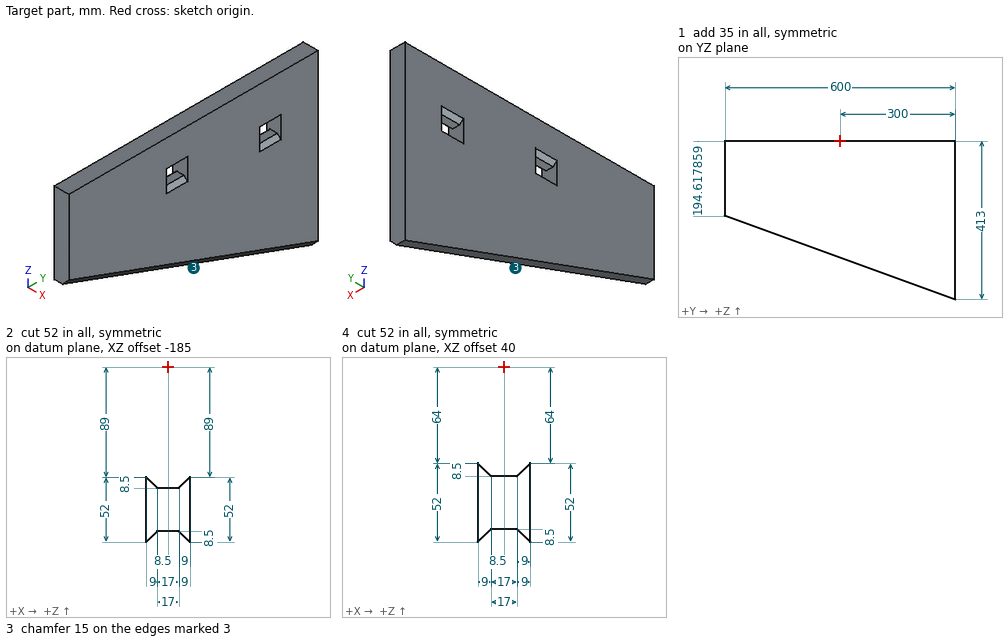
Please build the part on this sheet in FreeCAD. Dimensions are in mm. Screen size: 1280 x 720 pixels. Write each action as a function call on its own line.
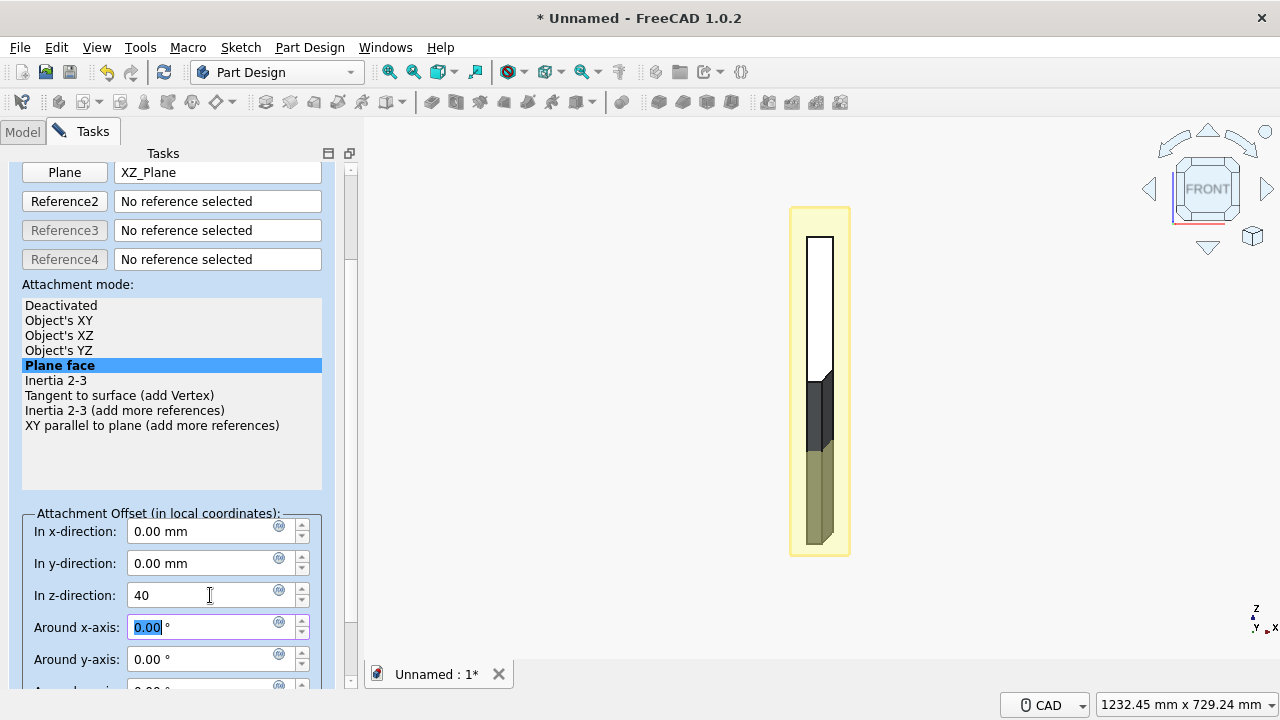
scroll(351, 426, up, 3)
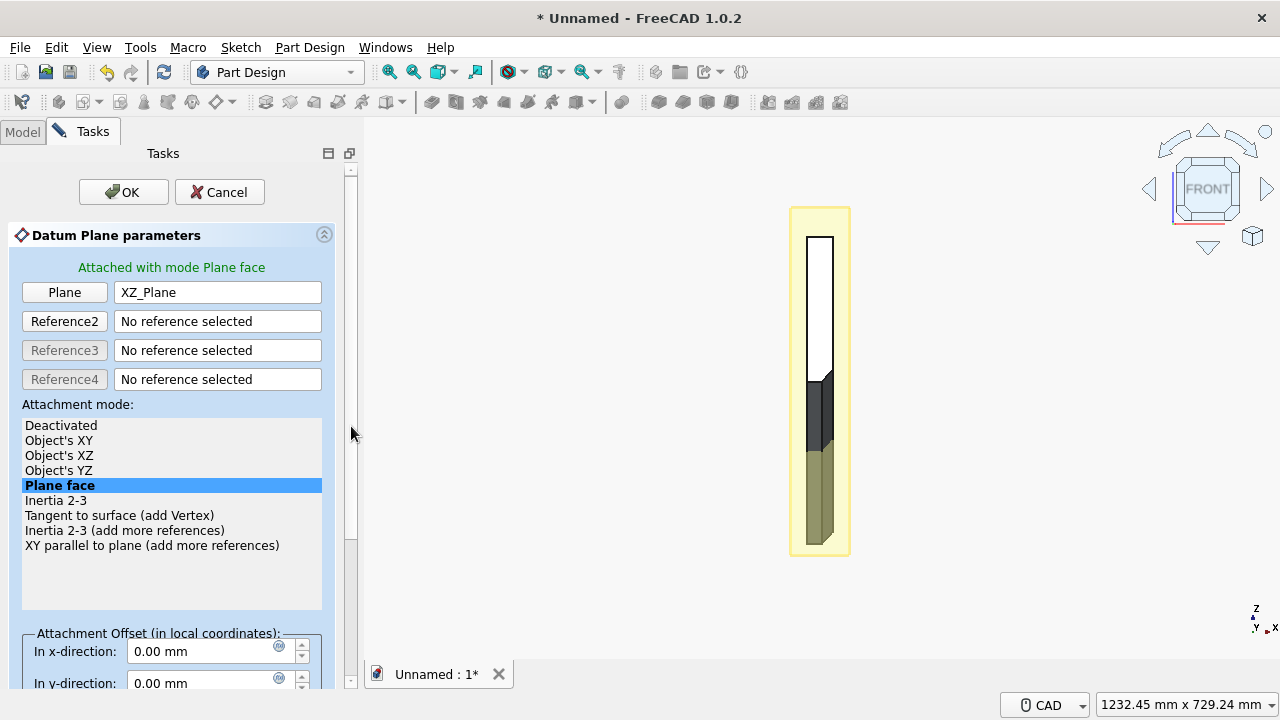
click(124, 192)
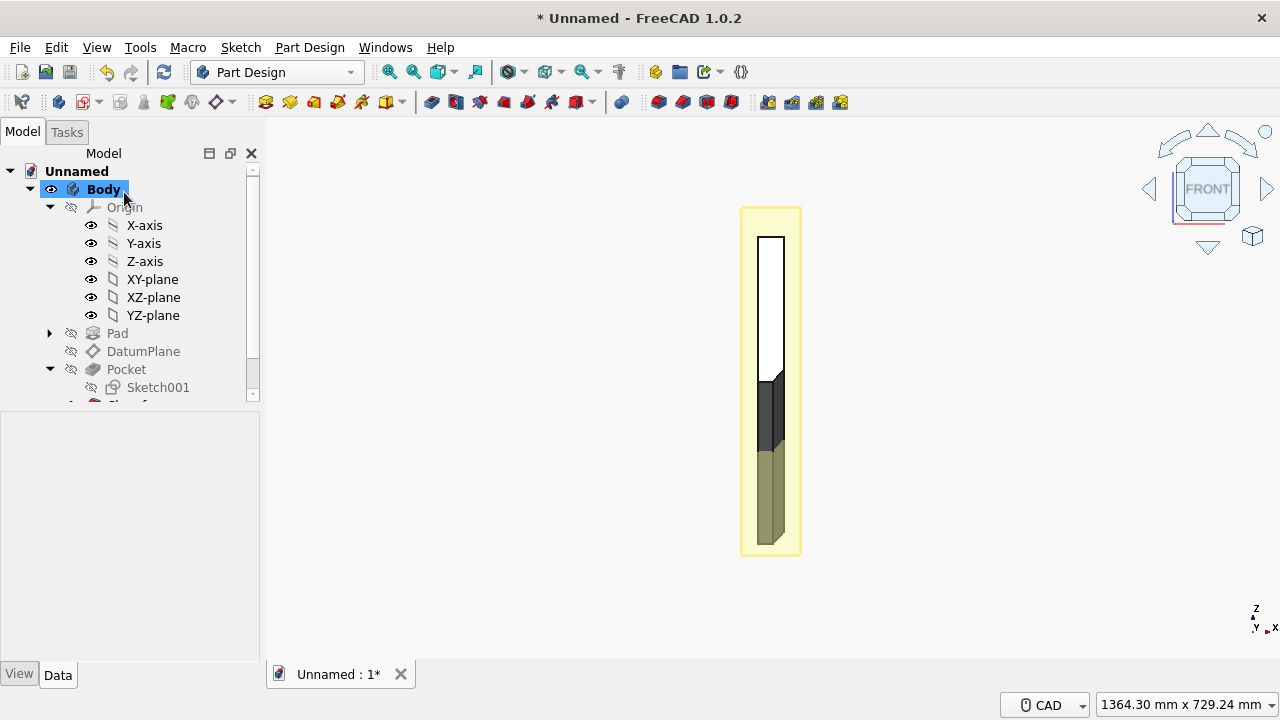
scroll(100, 275, down, 3)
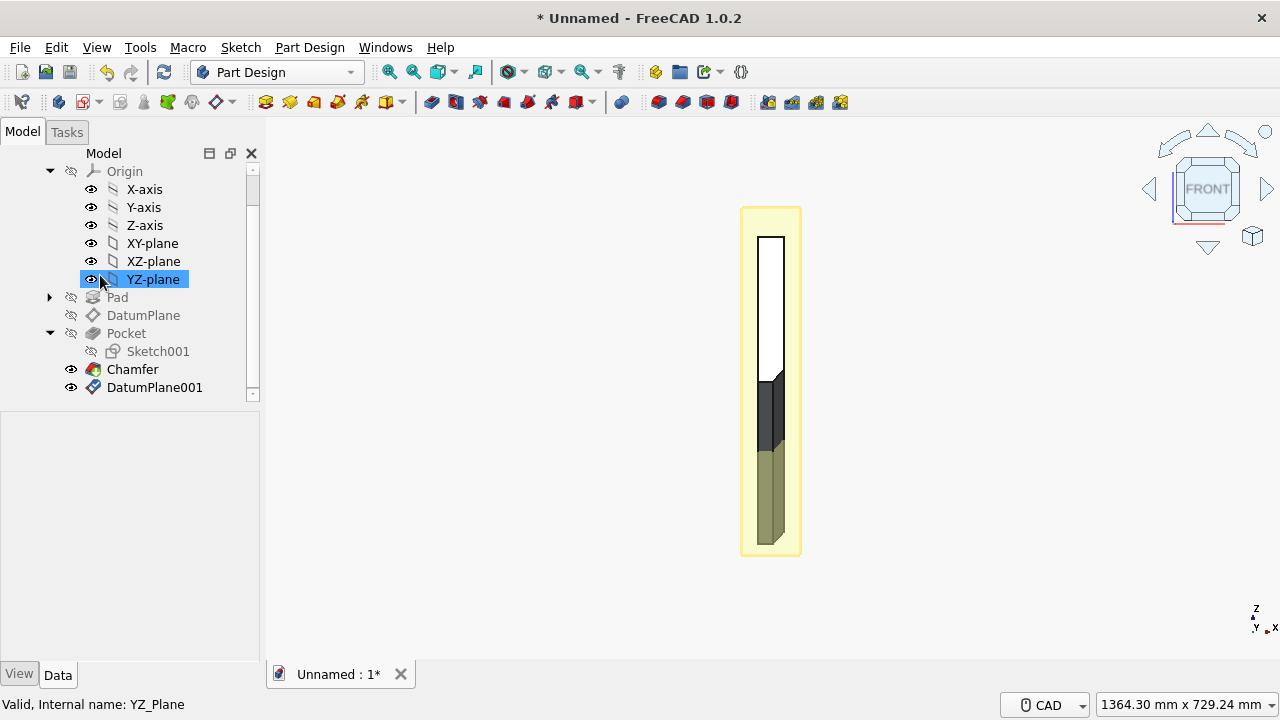
click(116, 387)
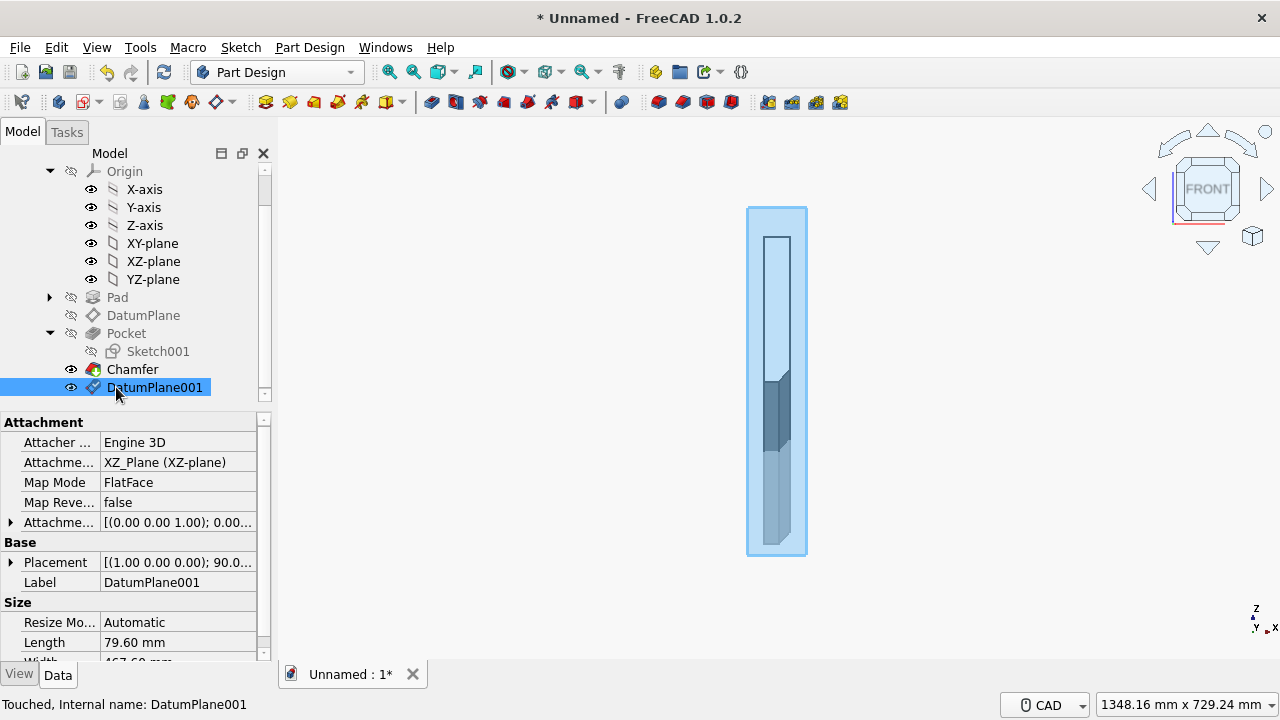
click(84, 102)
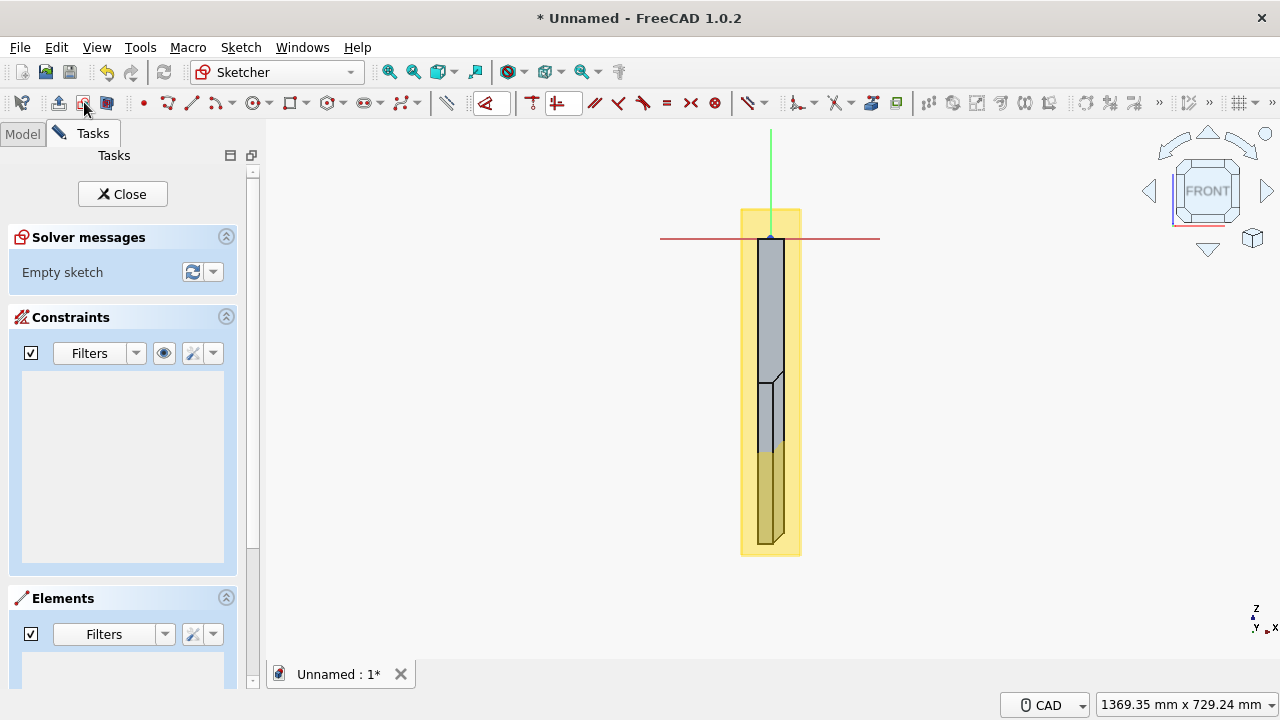
key(q)
key(s)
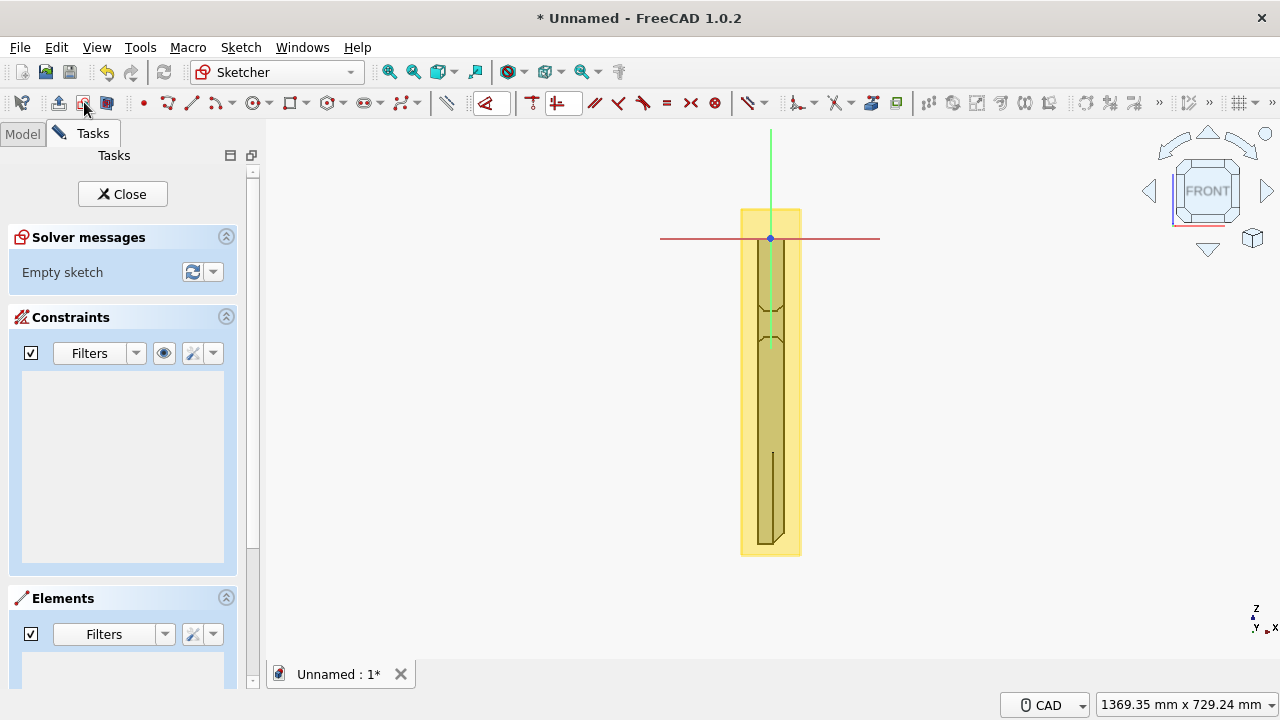
scroll(792, 246, up, 7)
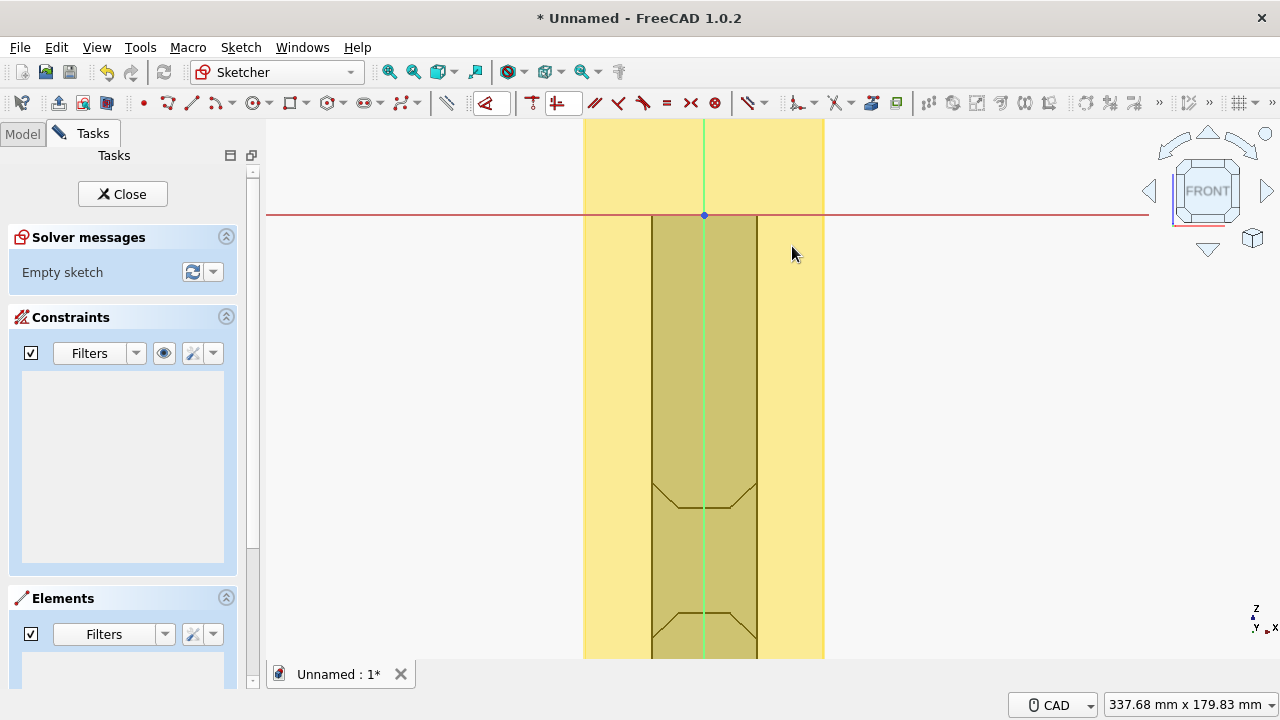
key(g)
key(m)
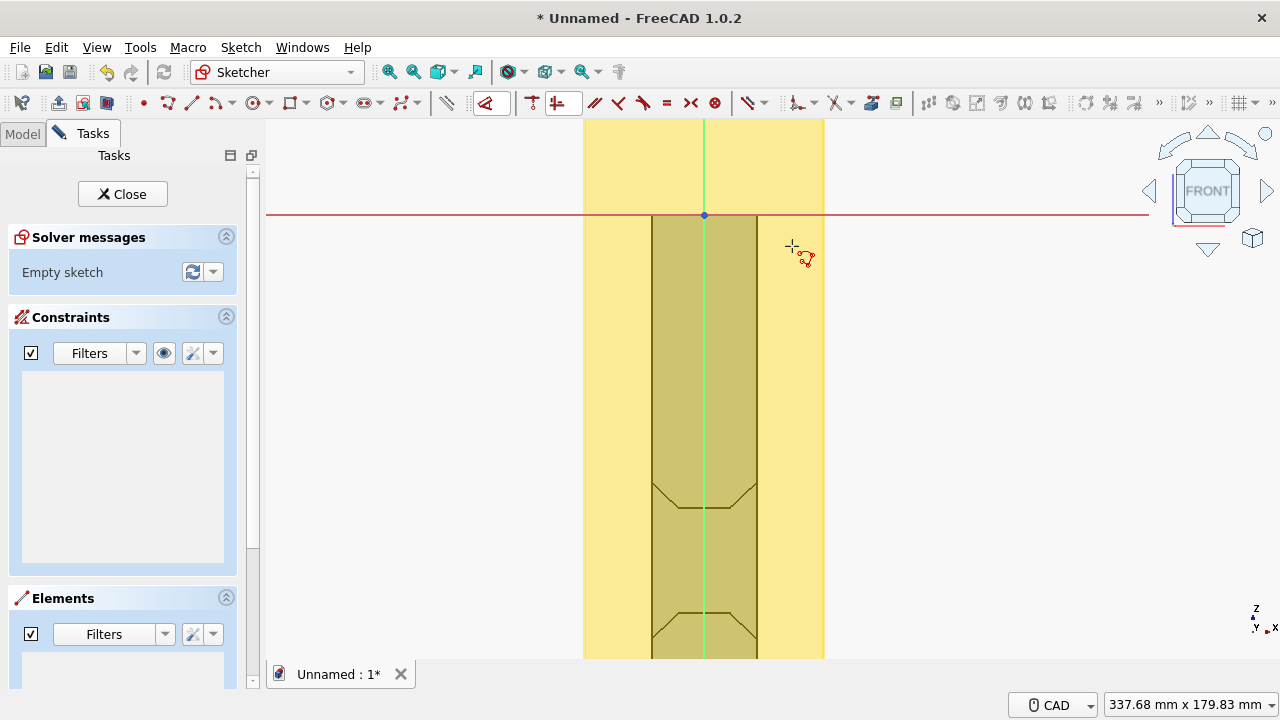
click(652, 408)
click(679, 433)
click(730, 433)
click(757, 408)
click(757, 564)
click(730, 538)
click(679, 538)
click(652, 564)
click(652, 409)
key(Escape)
key(Escape)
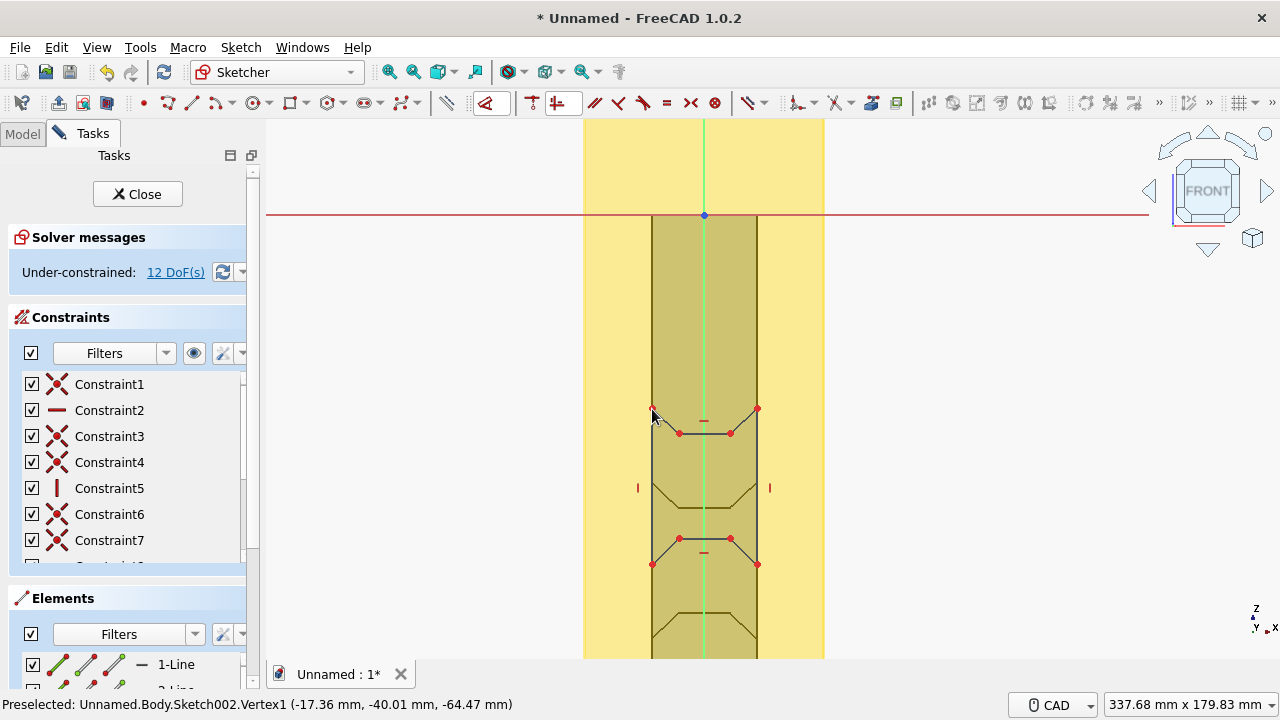
scroll(694, 434, up, 2)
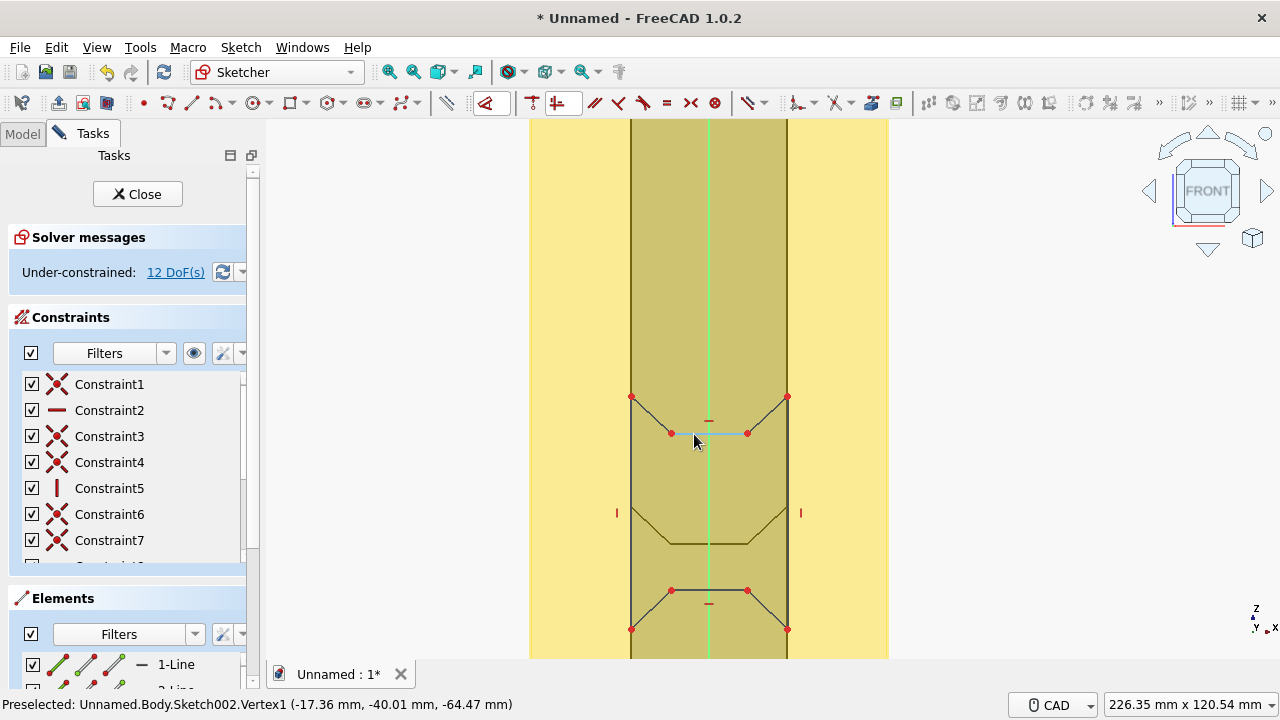
click(694, 434)